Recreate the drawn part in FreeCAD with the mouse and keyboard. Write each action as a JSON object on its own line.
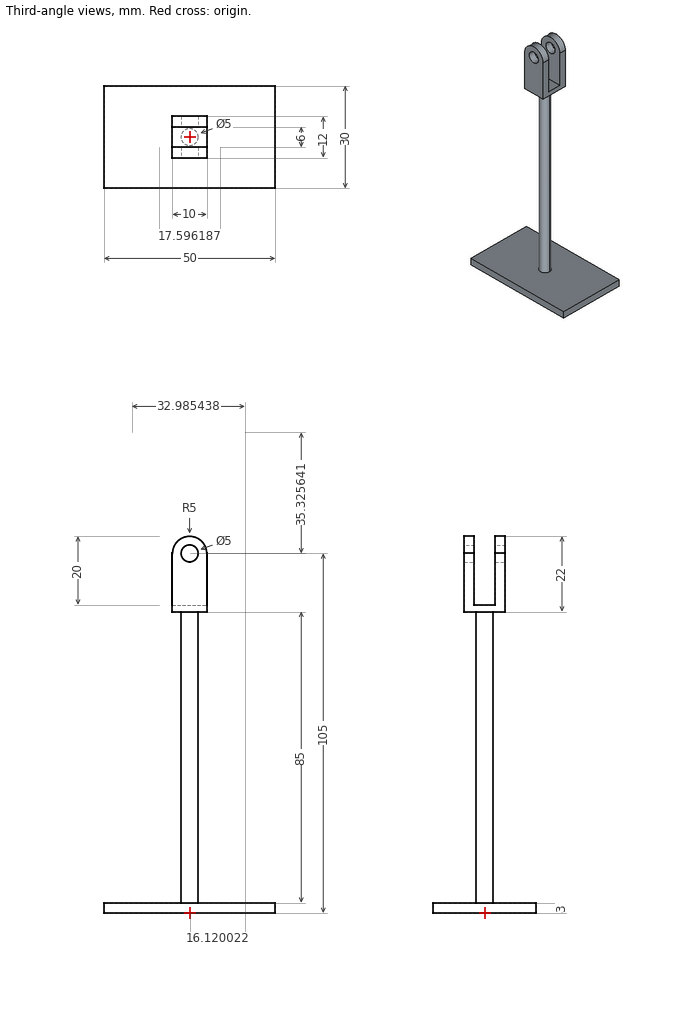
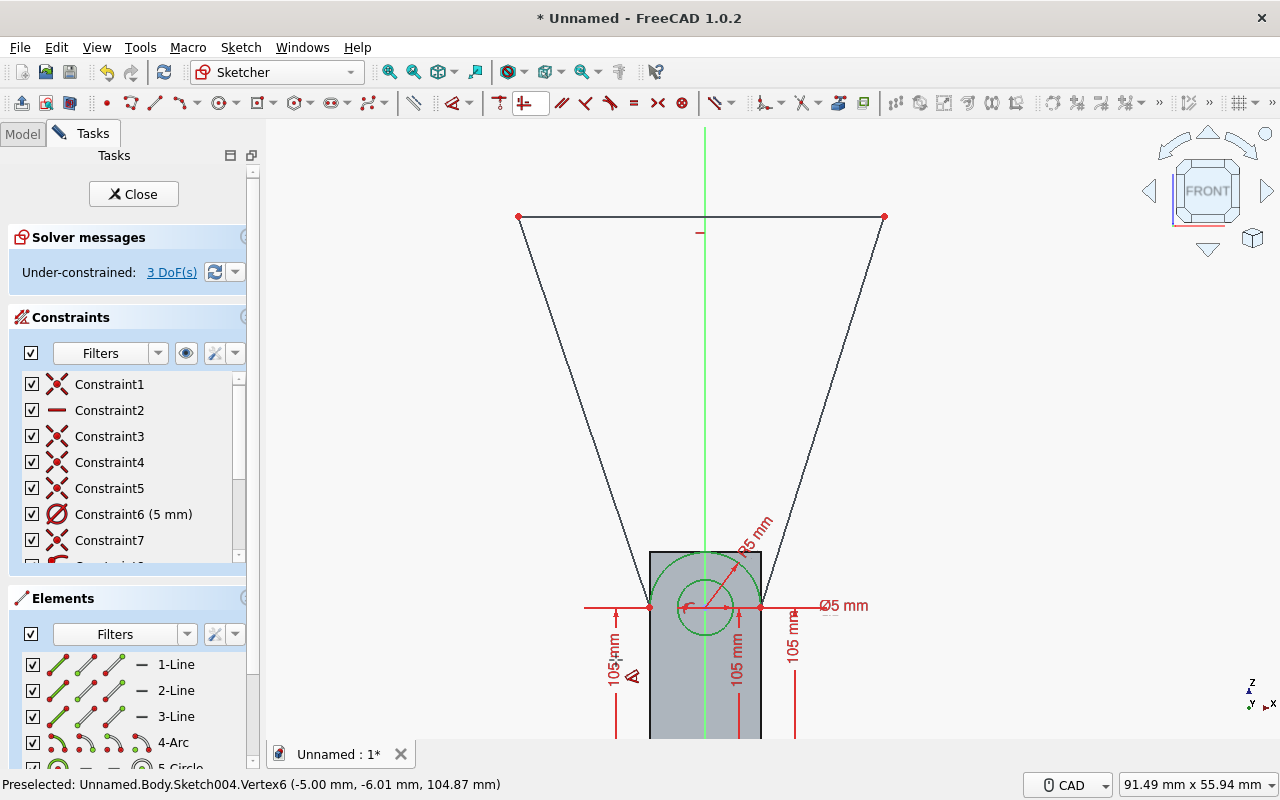
{"action": "left_click", "coordinate": [774, 217]}
{"action": "left_click", "coordinate": [617, 183]}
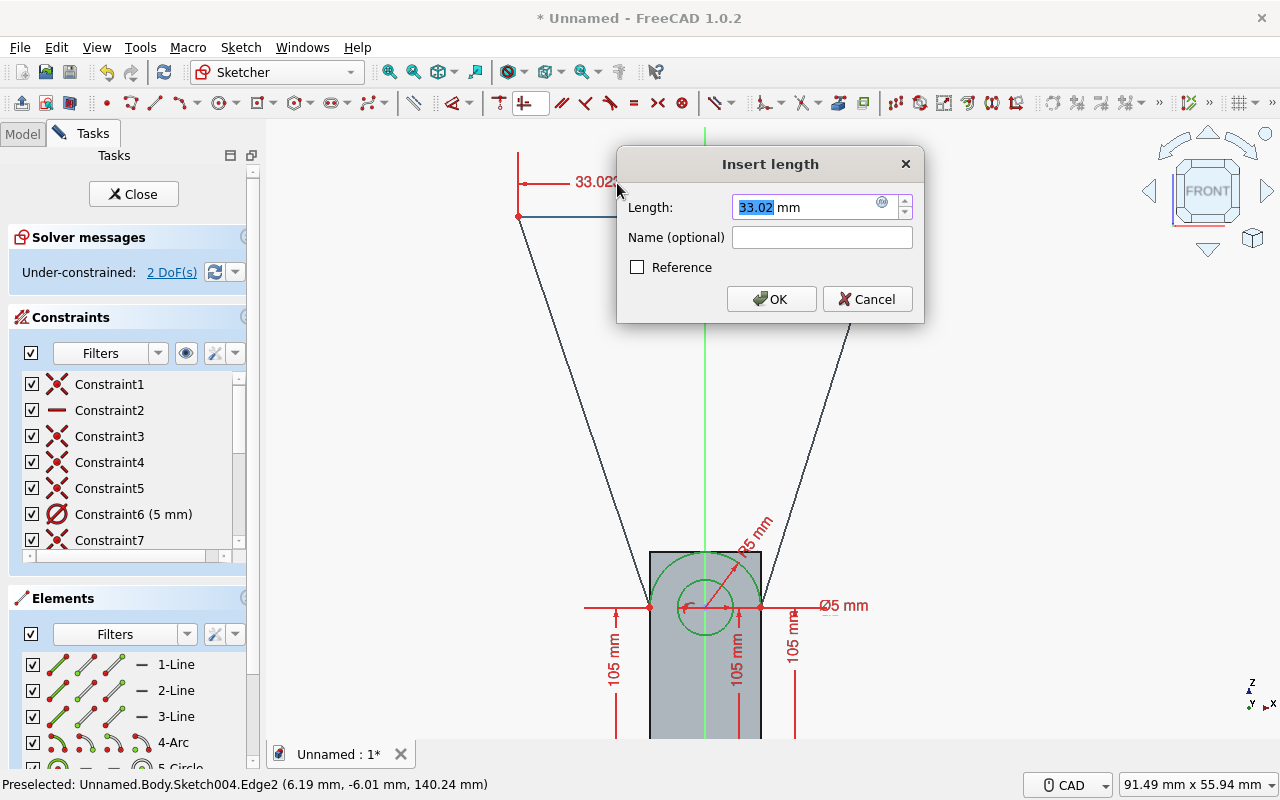
{"action": "type", "text": "32.985438"}
{"action": "key", "text": "Return"}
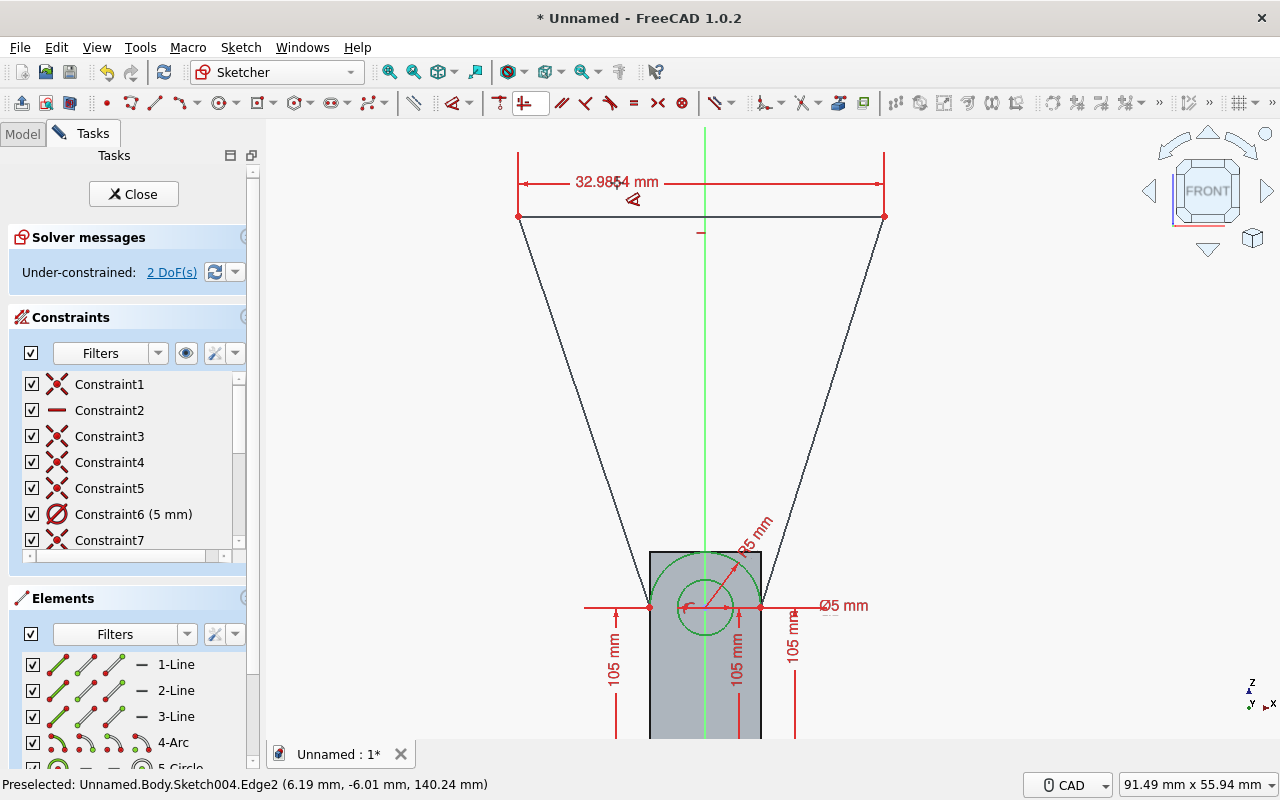
{"action": "left_click", "coordinate": [884, 217]}
{"action": "left_click", "coordinate": [795, 183]}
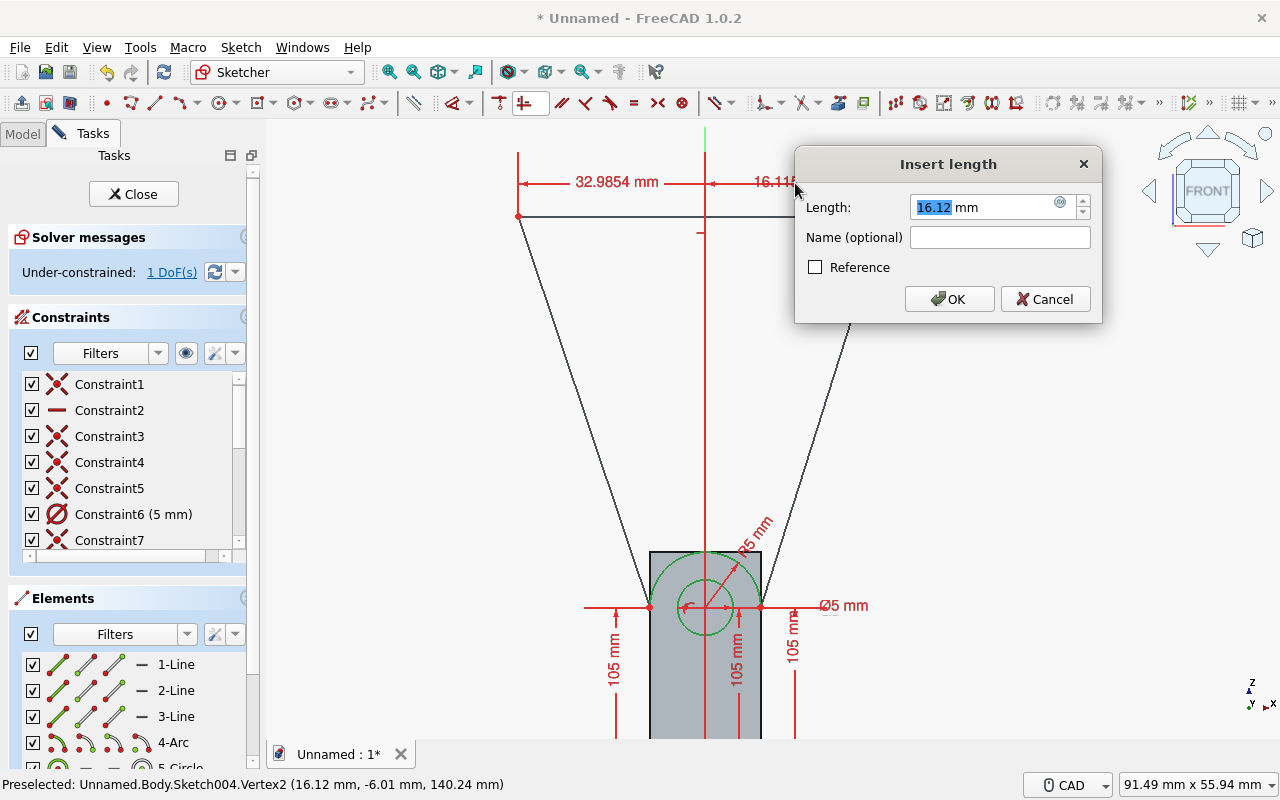
{"action": "type", "text": "16.120022"}
{"action": "key", "text": "Return"}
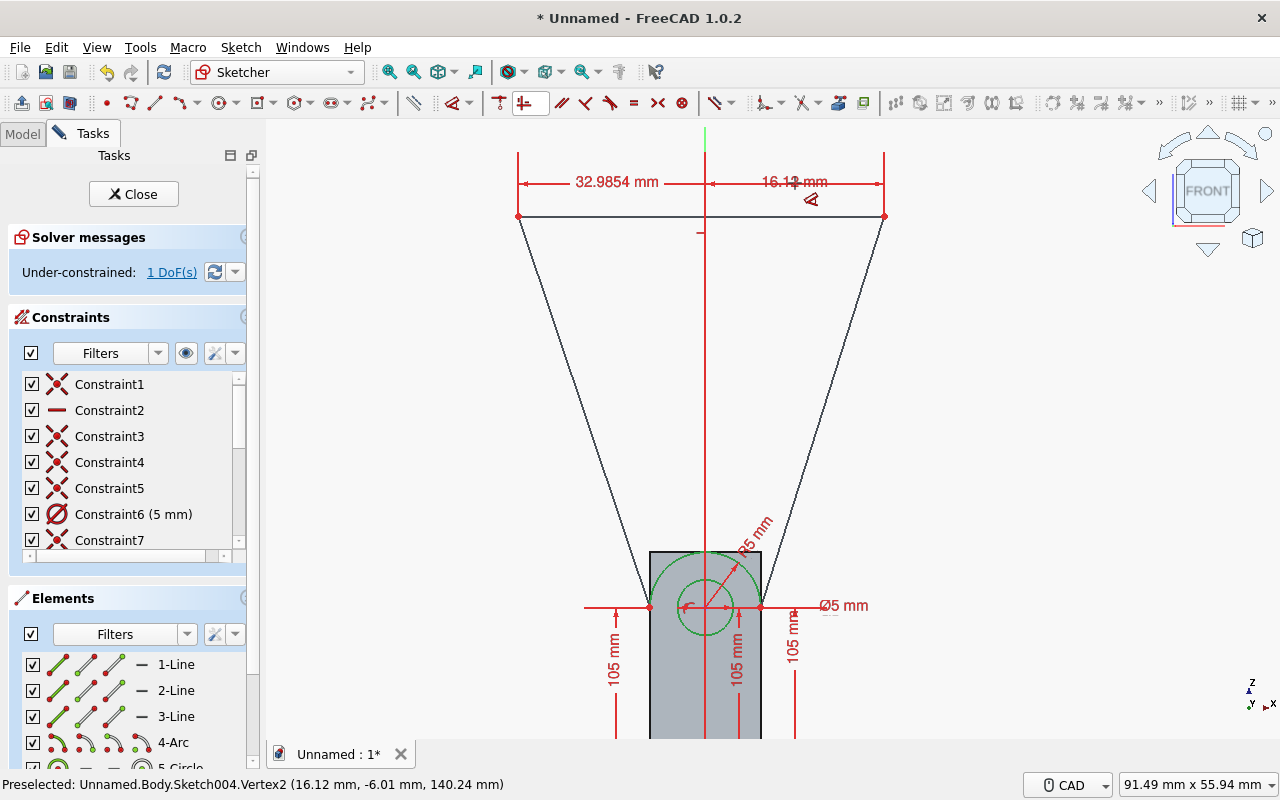
{"action": "left_click", "coordinate": [798, 490]}
{"action": "left_click", "coordinate": [918, 412]}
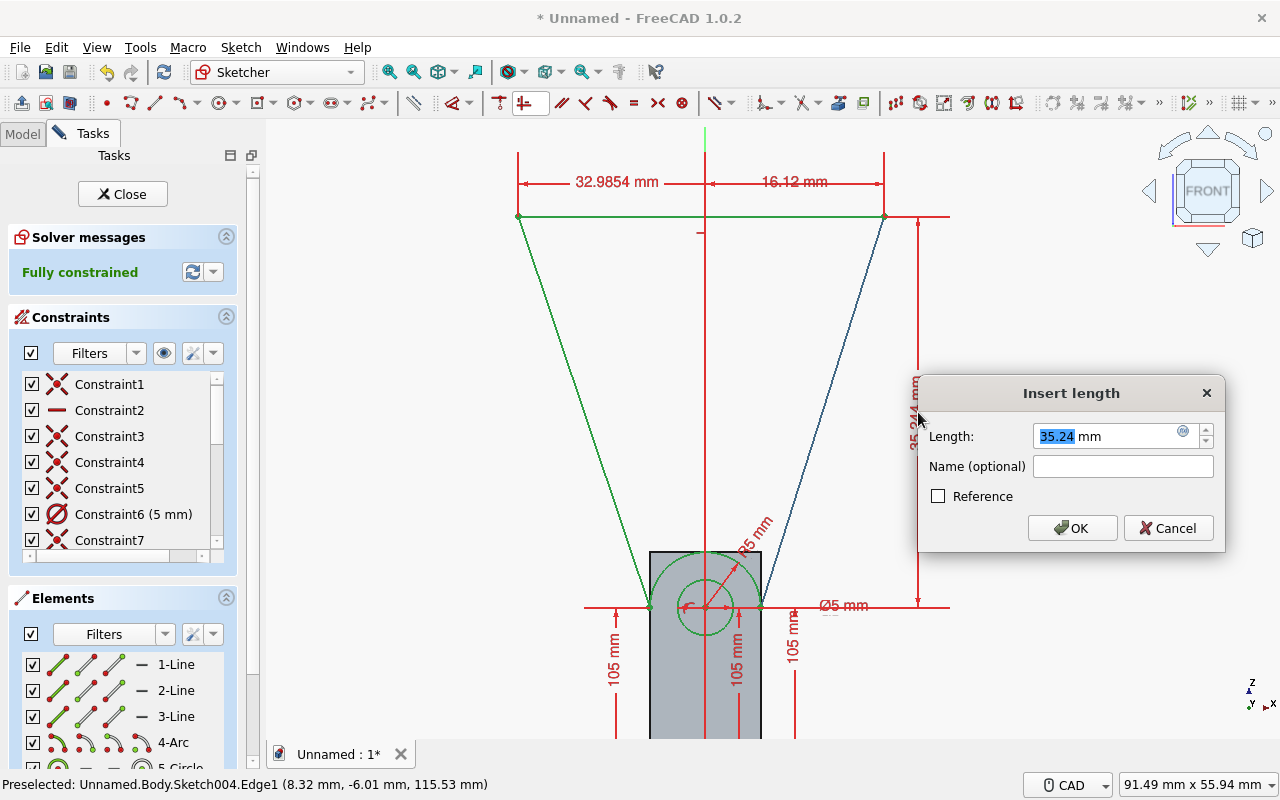
{"action": "type", "text": "35.325641"}
{"action": "key", "text": "Return"}
{"action": "key", "text": "Escape"}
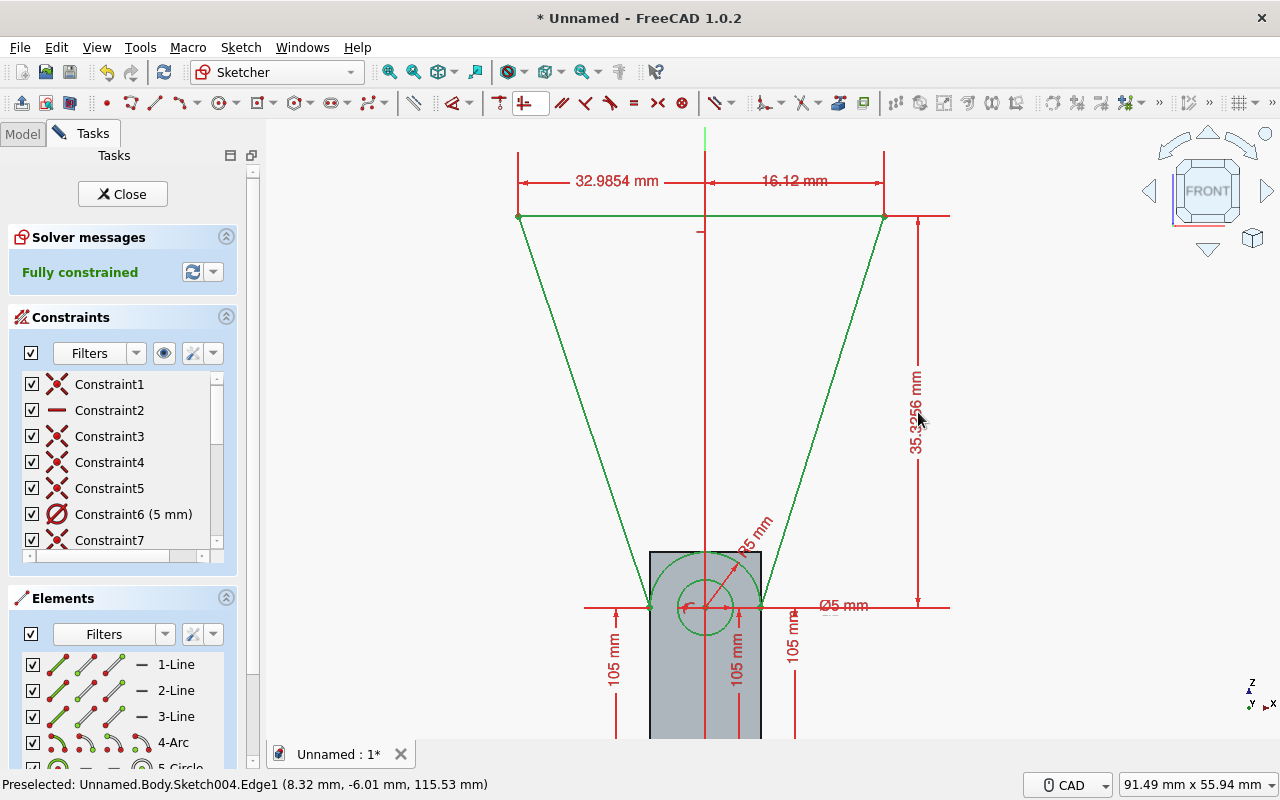
{"action": "left_click", "coordinate": [123, 194]}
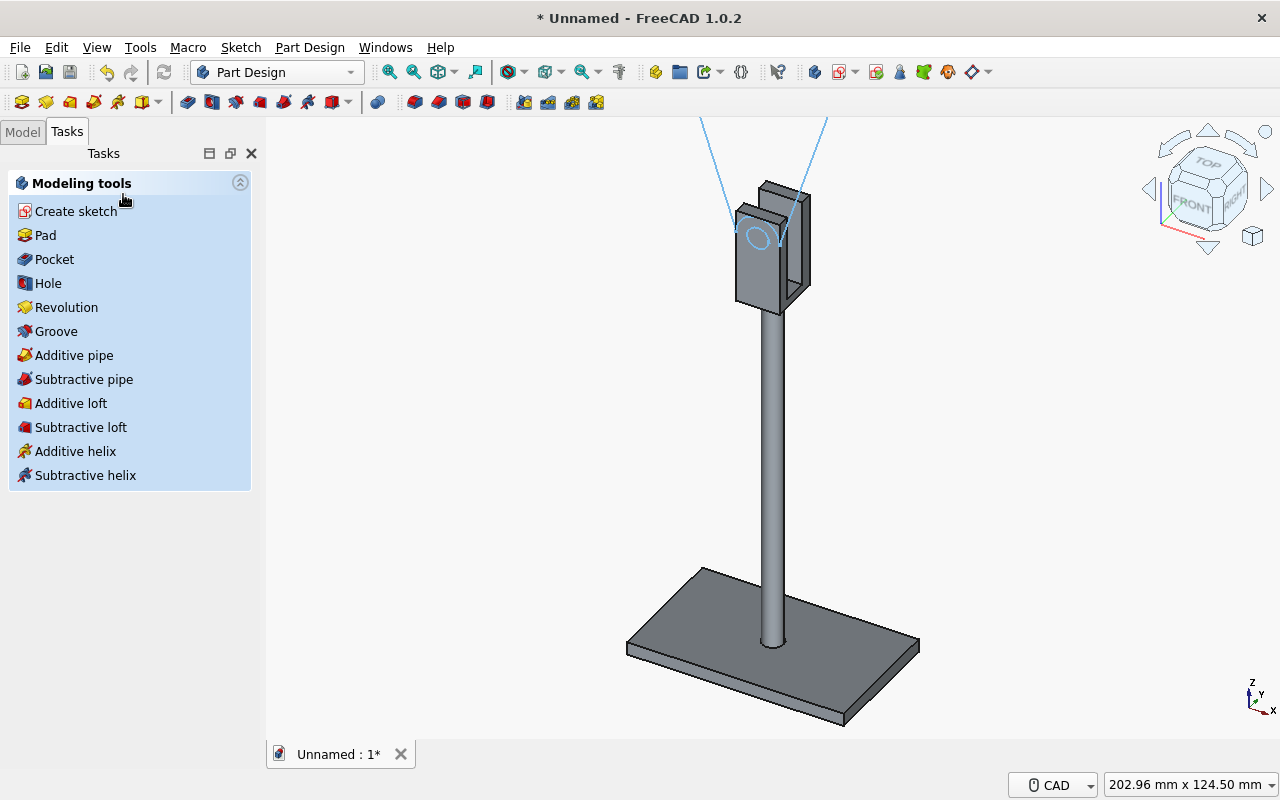
{"action": "left_click", "coordinate": [188, 102]}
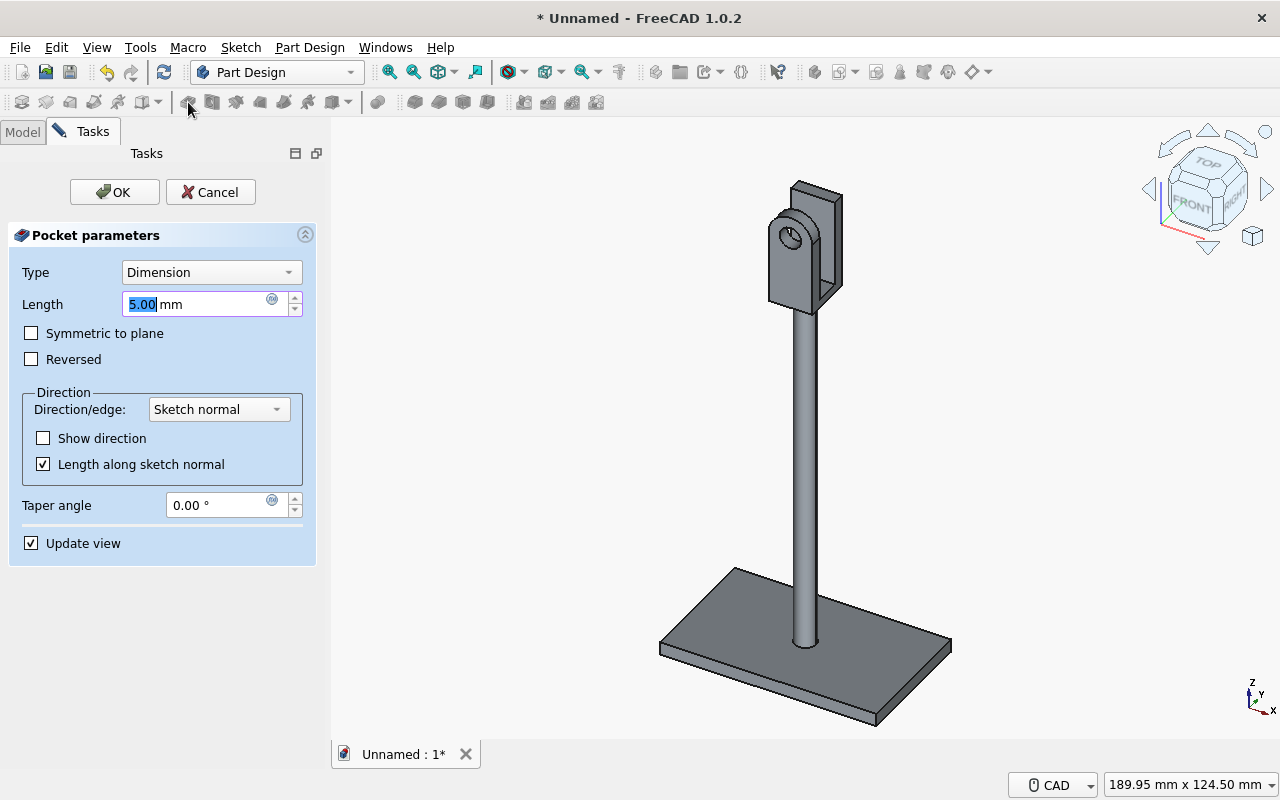
{"action": "left_click", "coordinate": [212, 272]}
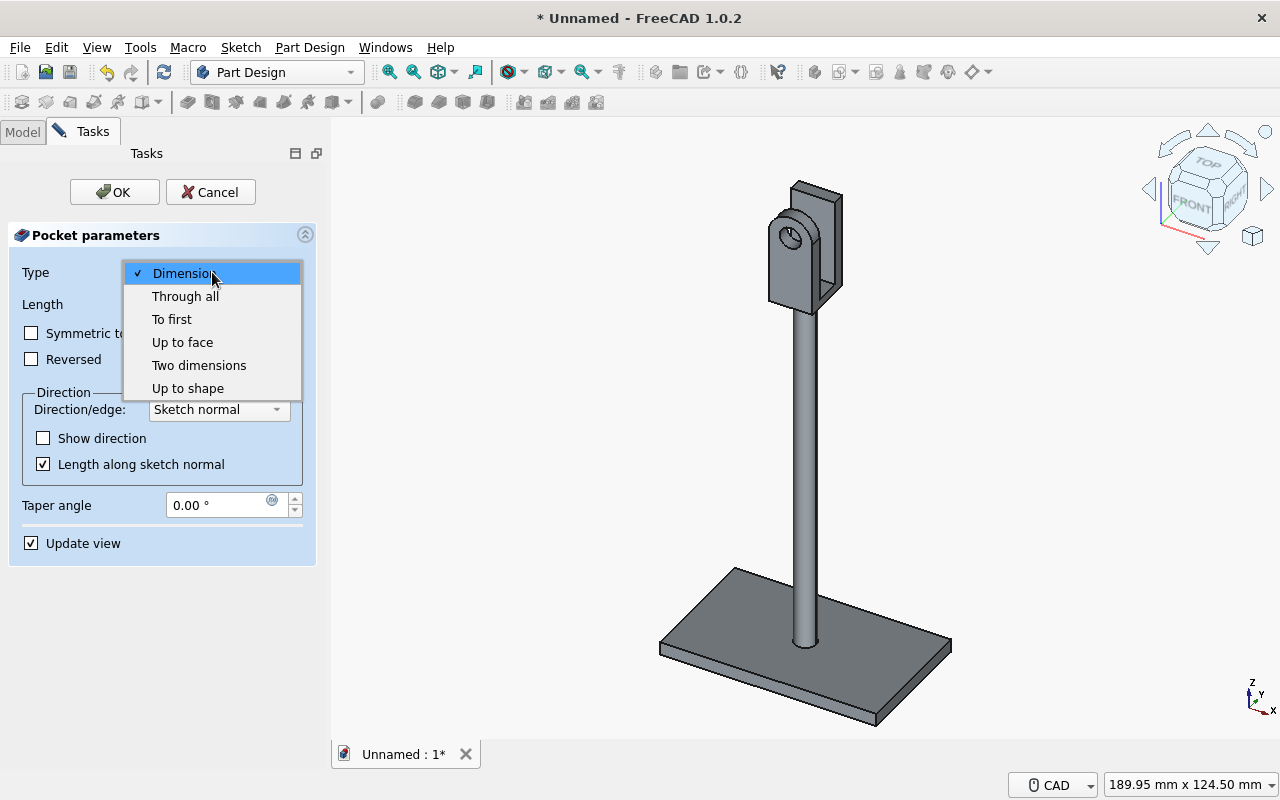
{"action": "left_click", "coordinate": [212, 296]}